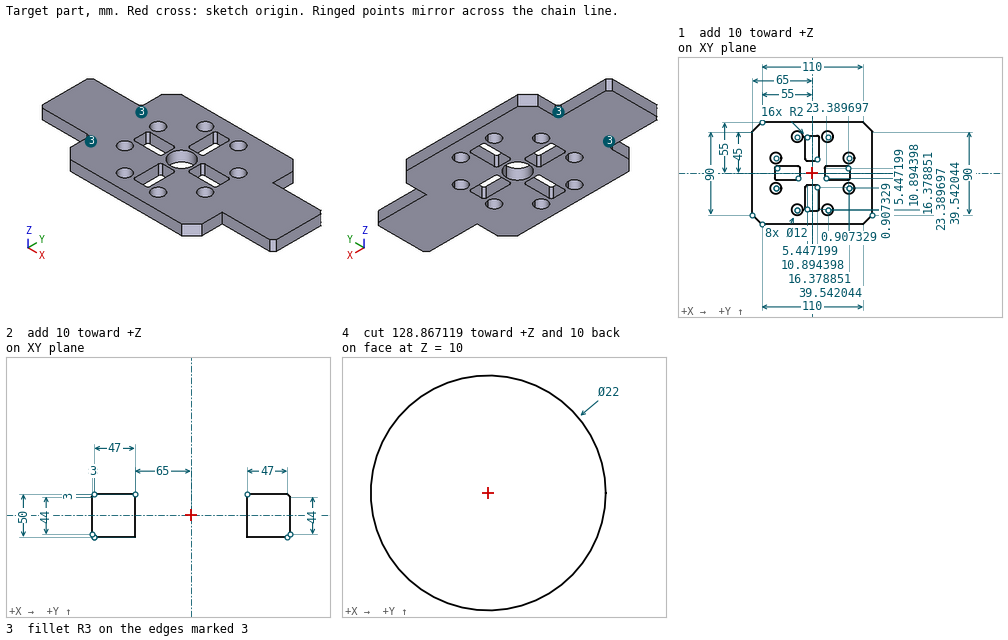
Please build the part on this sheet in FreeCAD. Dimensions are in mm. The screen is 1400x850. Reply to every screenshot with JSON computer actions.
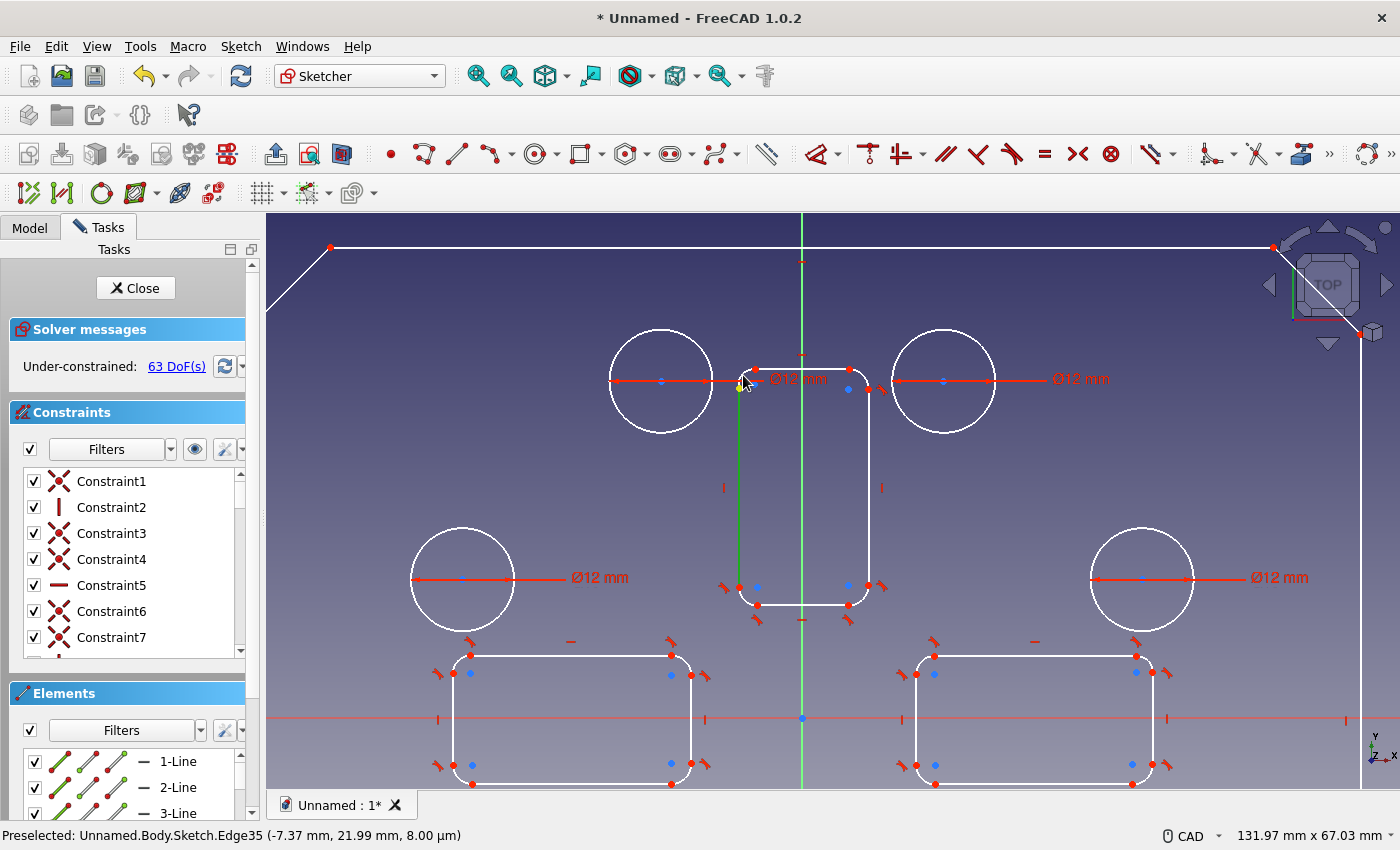
{"action": "left_click", "coordinate": [742, 375]}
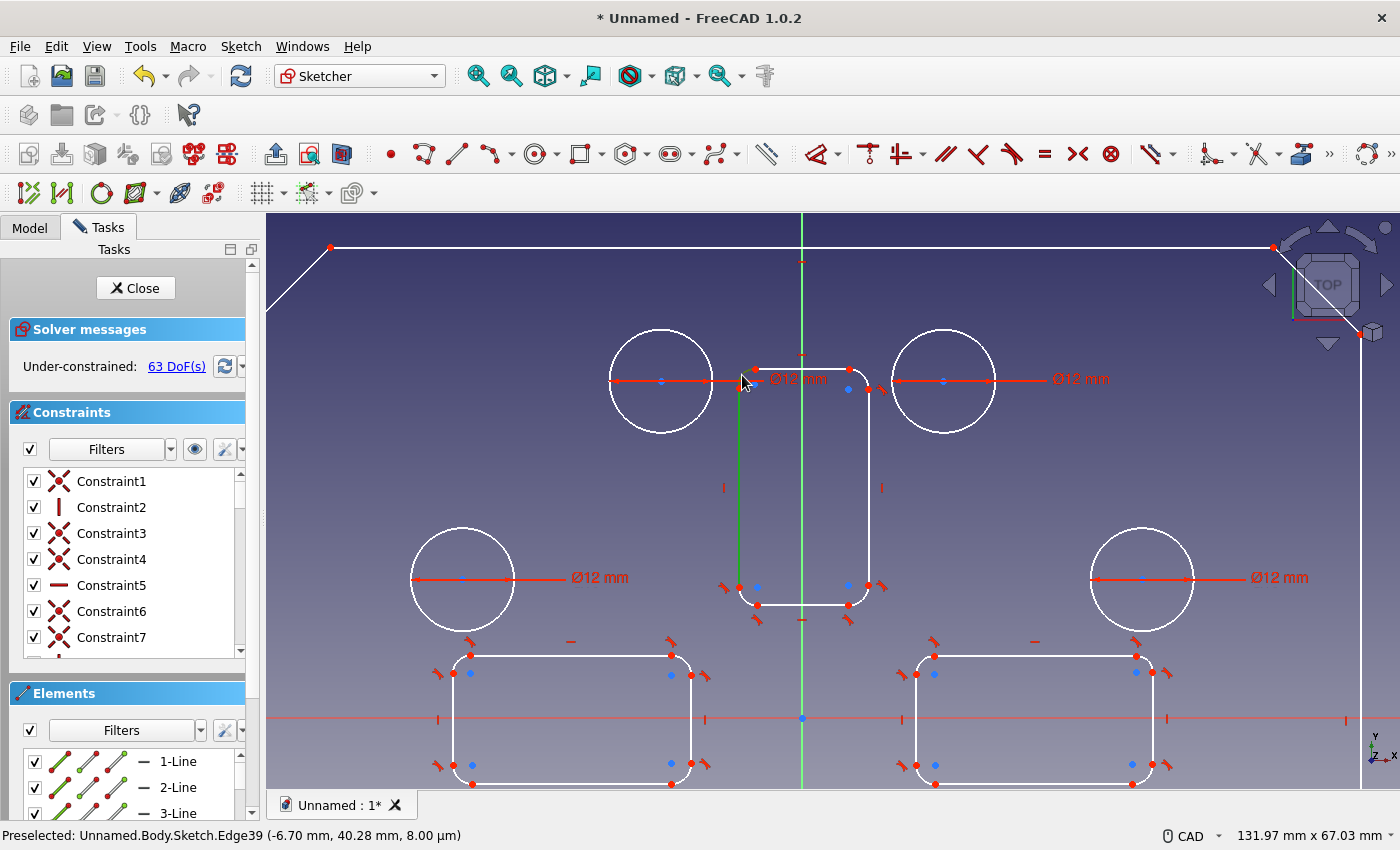
{"action": "left_click", "coordinate": [1012, 154]}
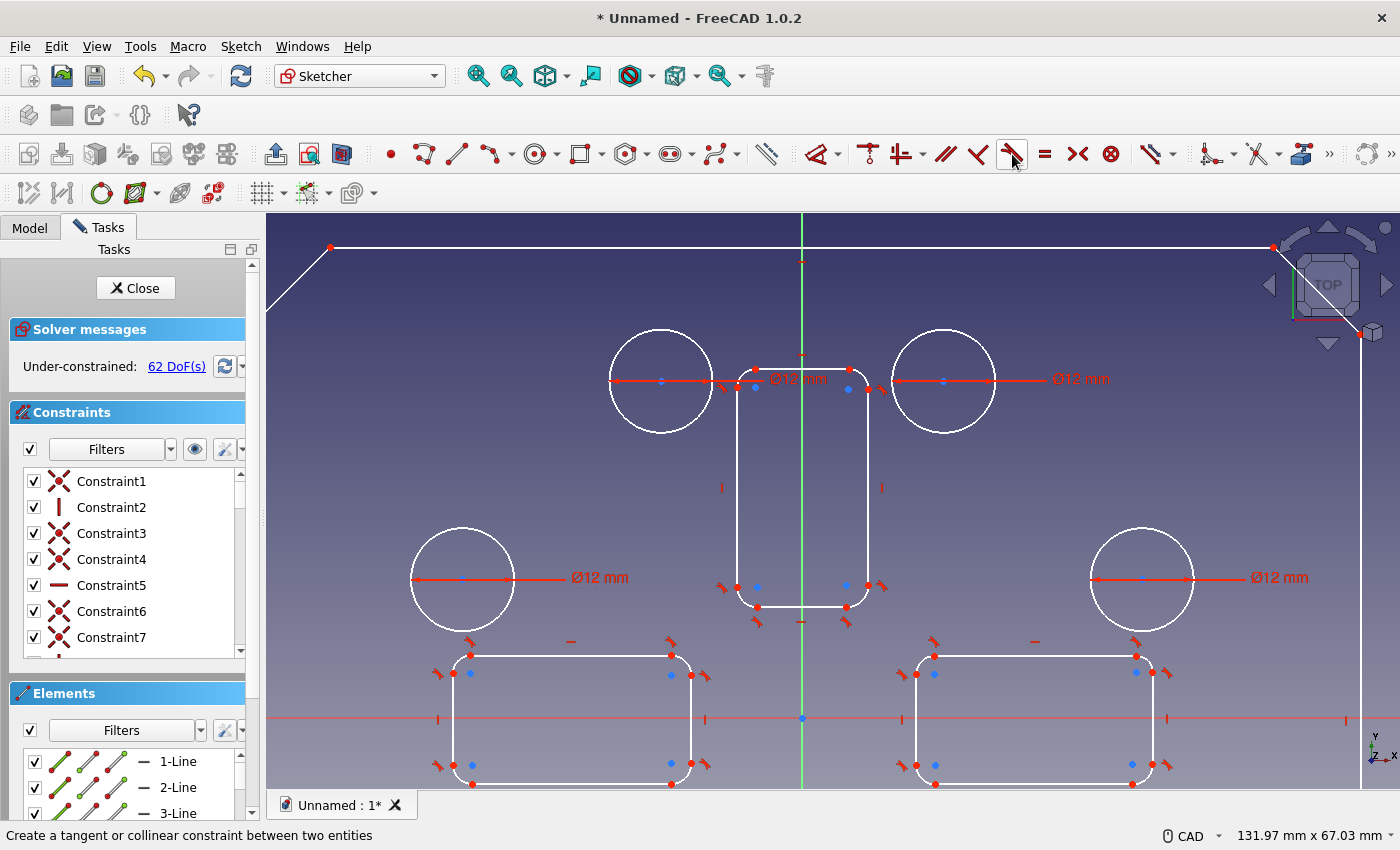
{"action": "left_click", "coordinate": [783, 369]}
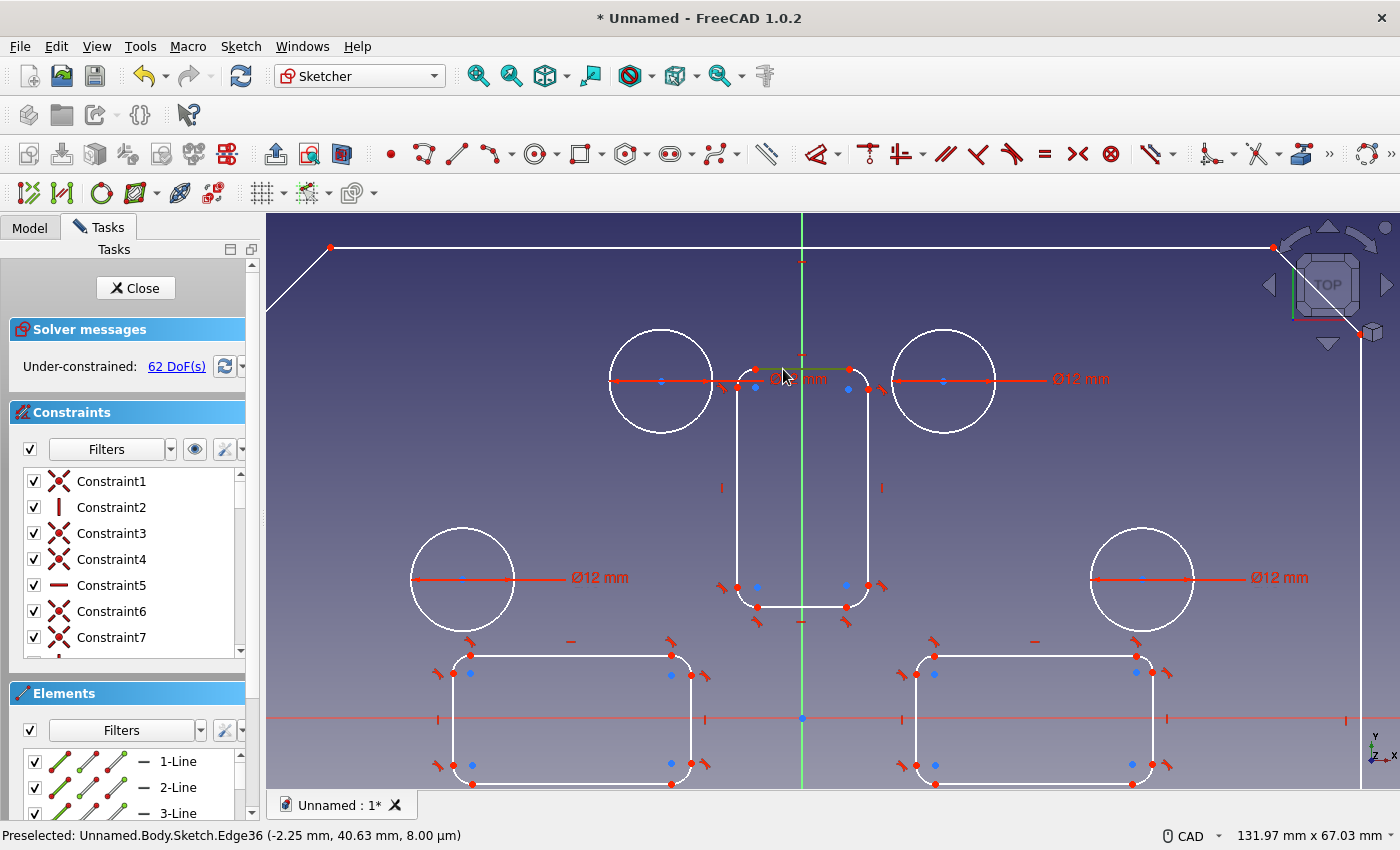
{"action": "left_click", "coordinate": [742, 375]}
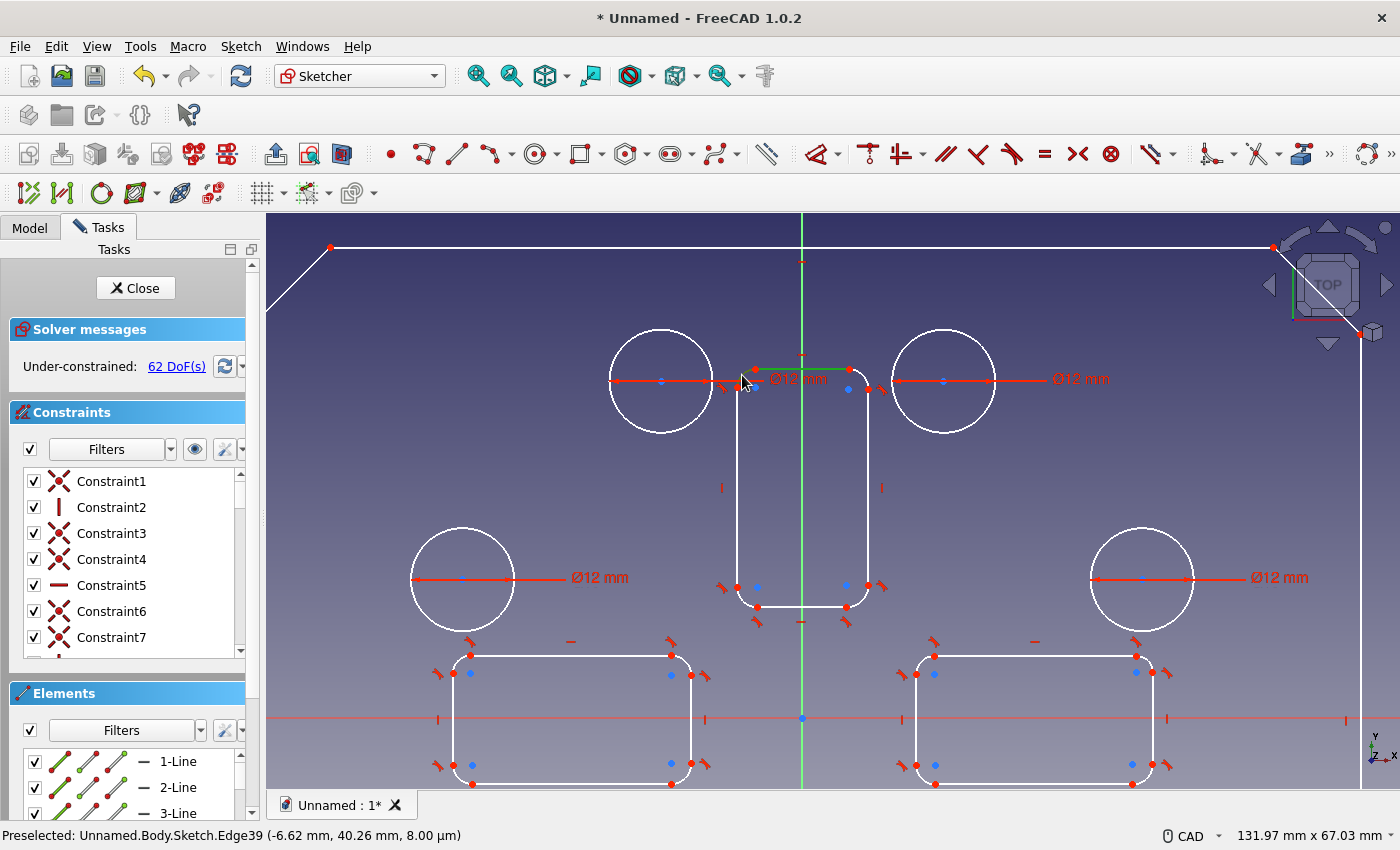
{"action": "left_click", "coordinate": [1012, 154]}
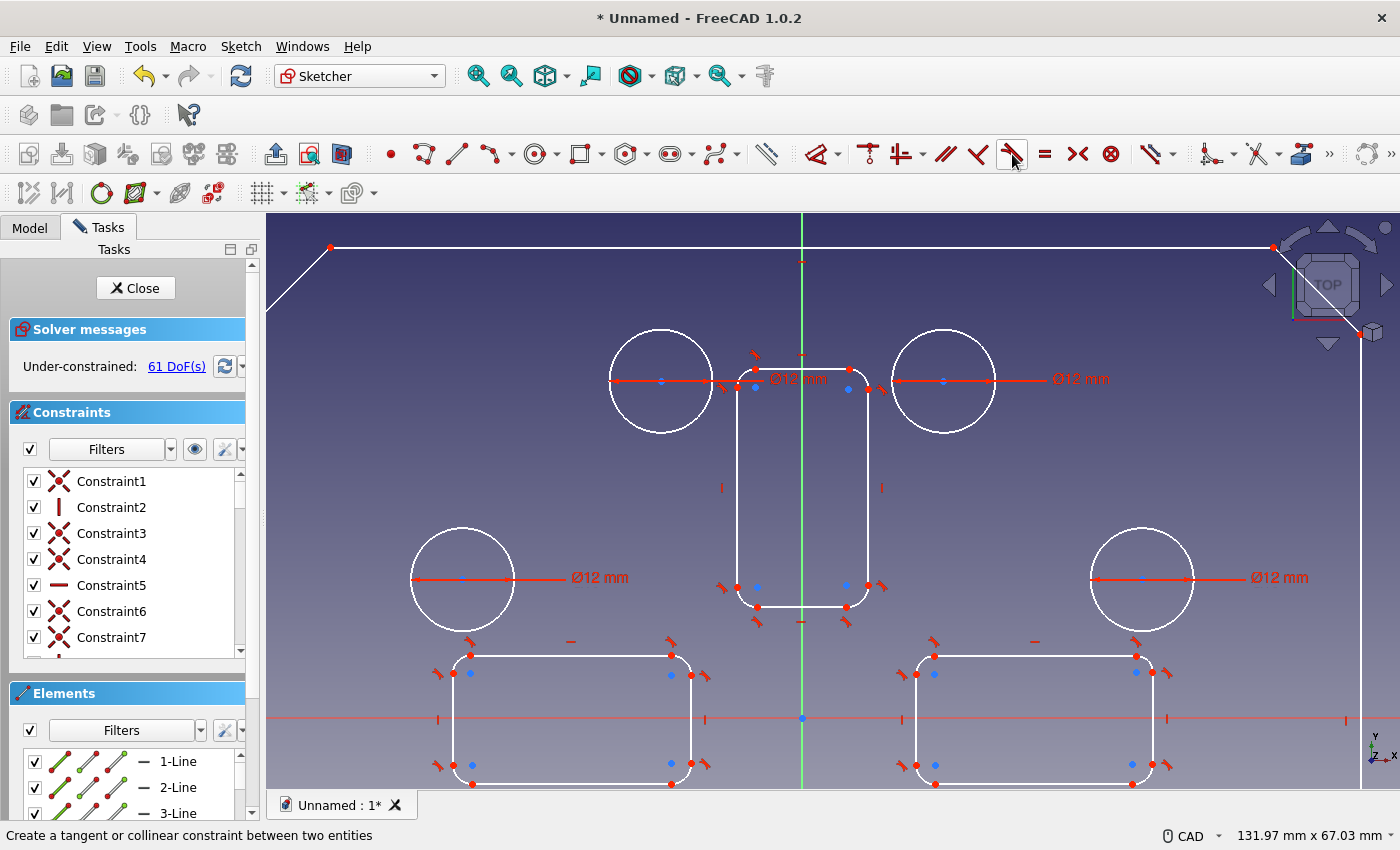
{"action": "left_click", "coordinate": [784, 369]}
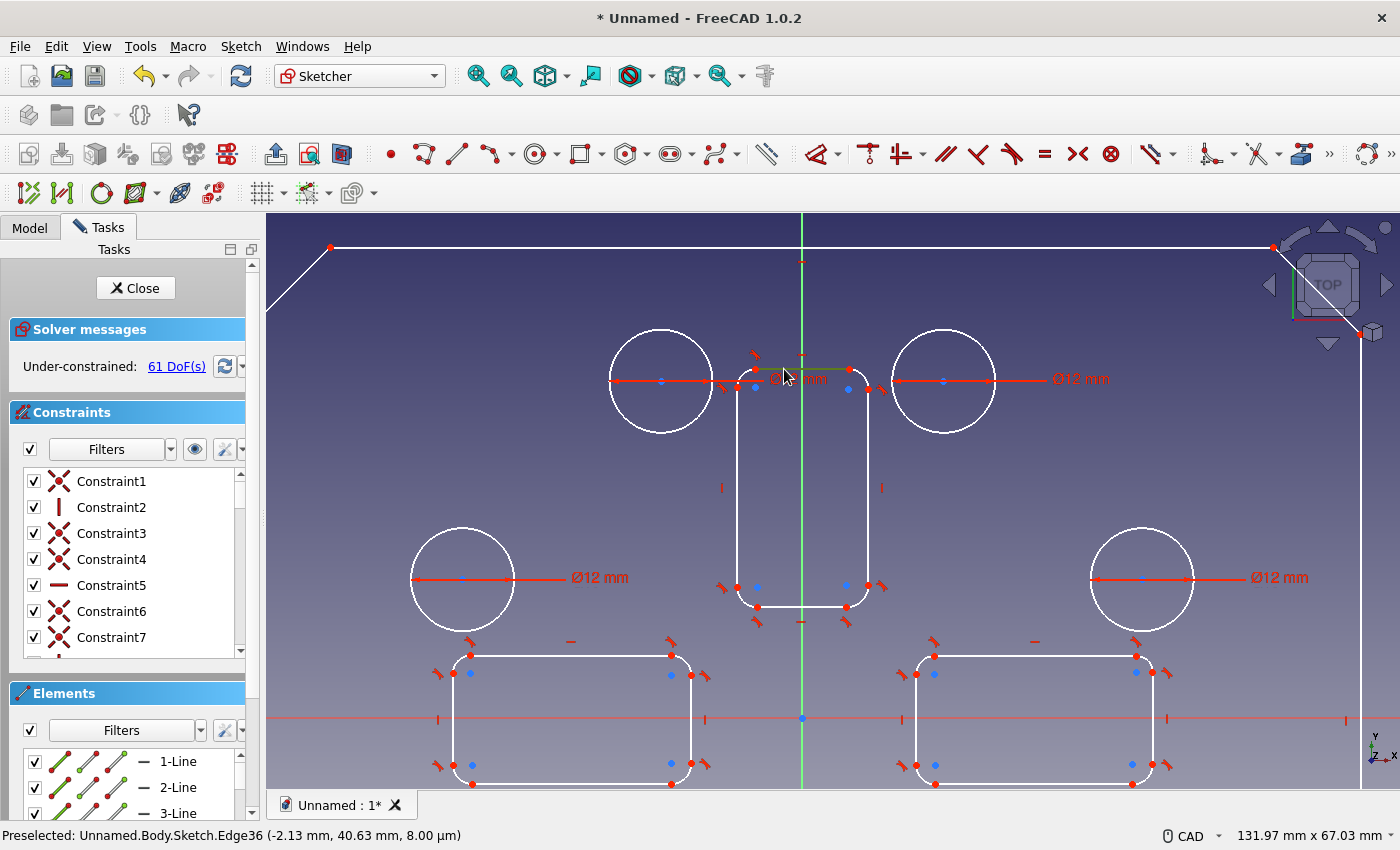
{"action": "scroll", "coordinate": [866, 380], "scroll_direction": "up", "scroll_amount": 3}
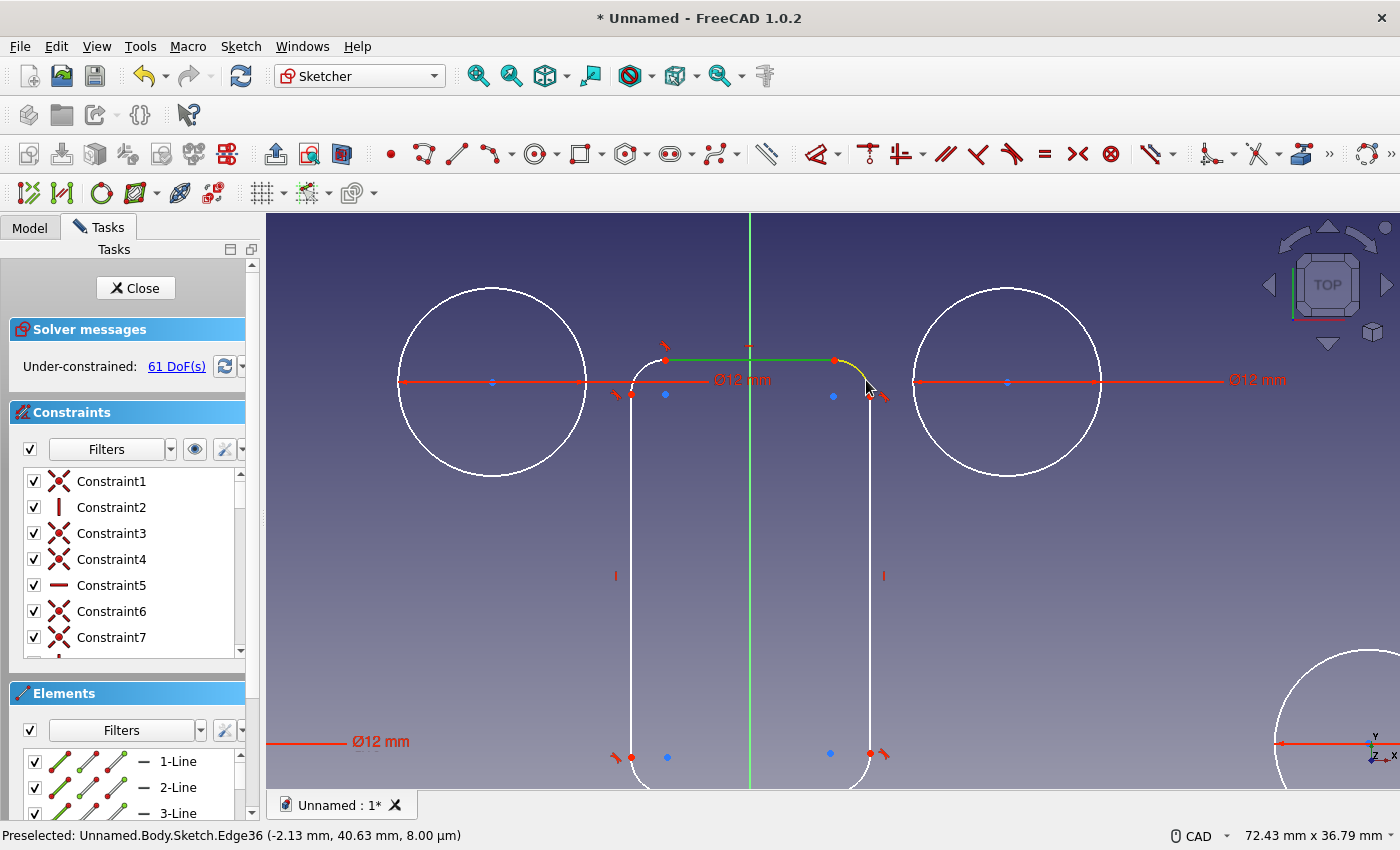
{"action": "left_click", "coordinate": [866, 380]}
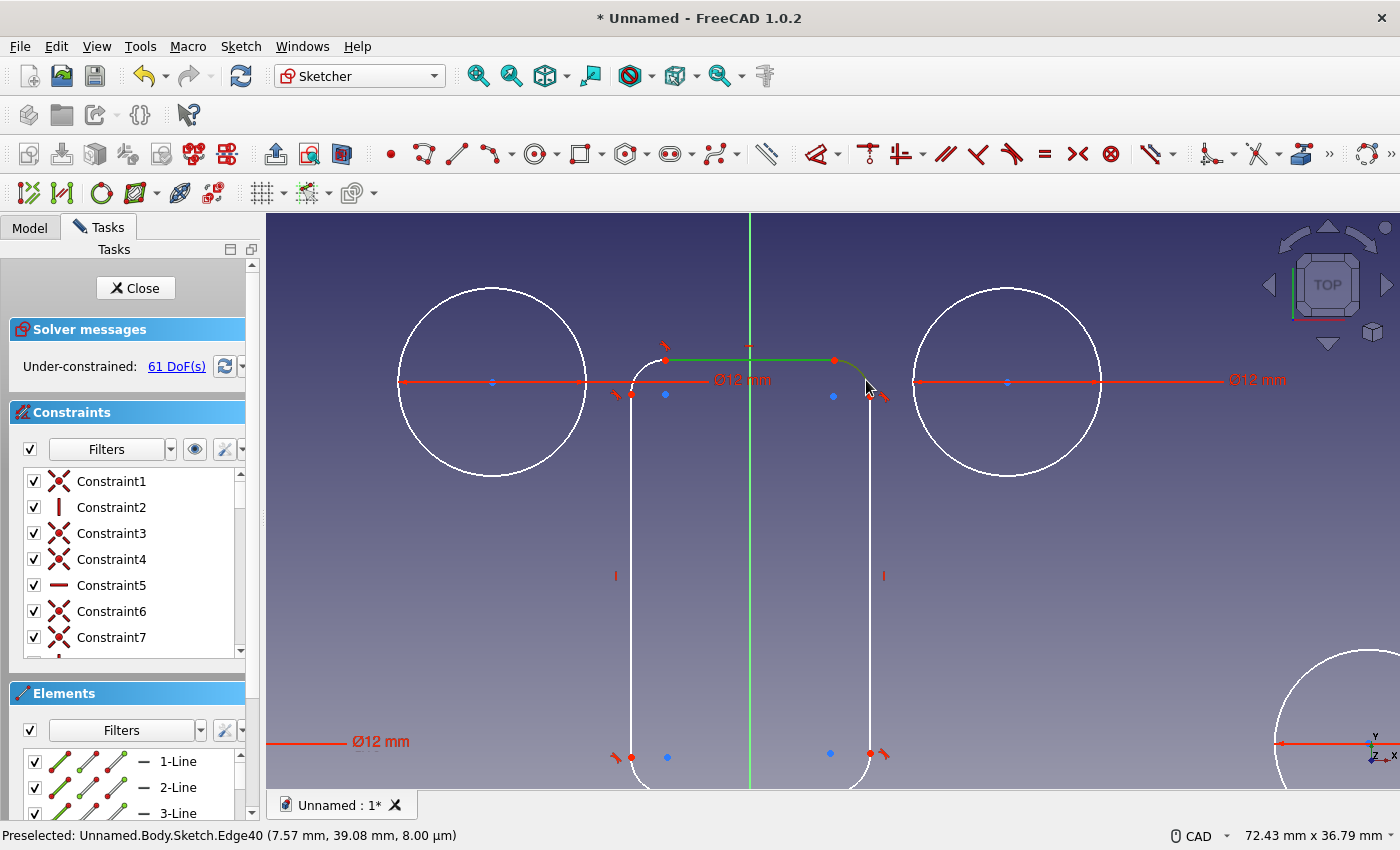
{"action": "left_click", "coordinate": [1012, 154]}